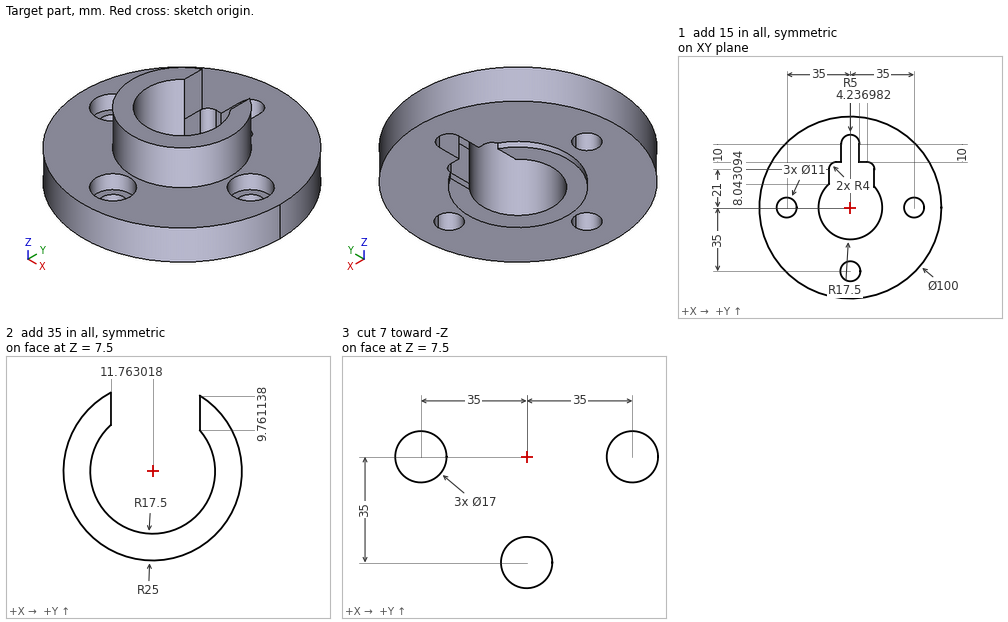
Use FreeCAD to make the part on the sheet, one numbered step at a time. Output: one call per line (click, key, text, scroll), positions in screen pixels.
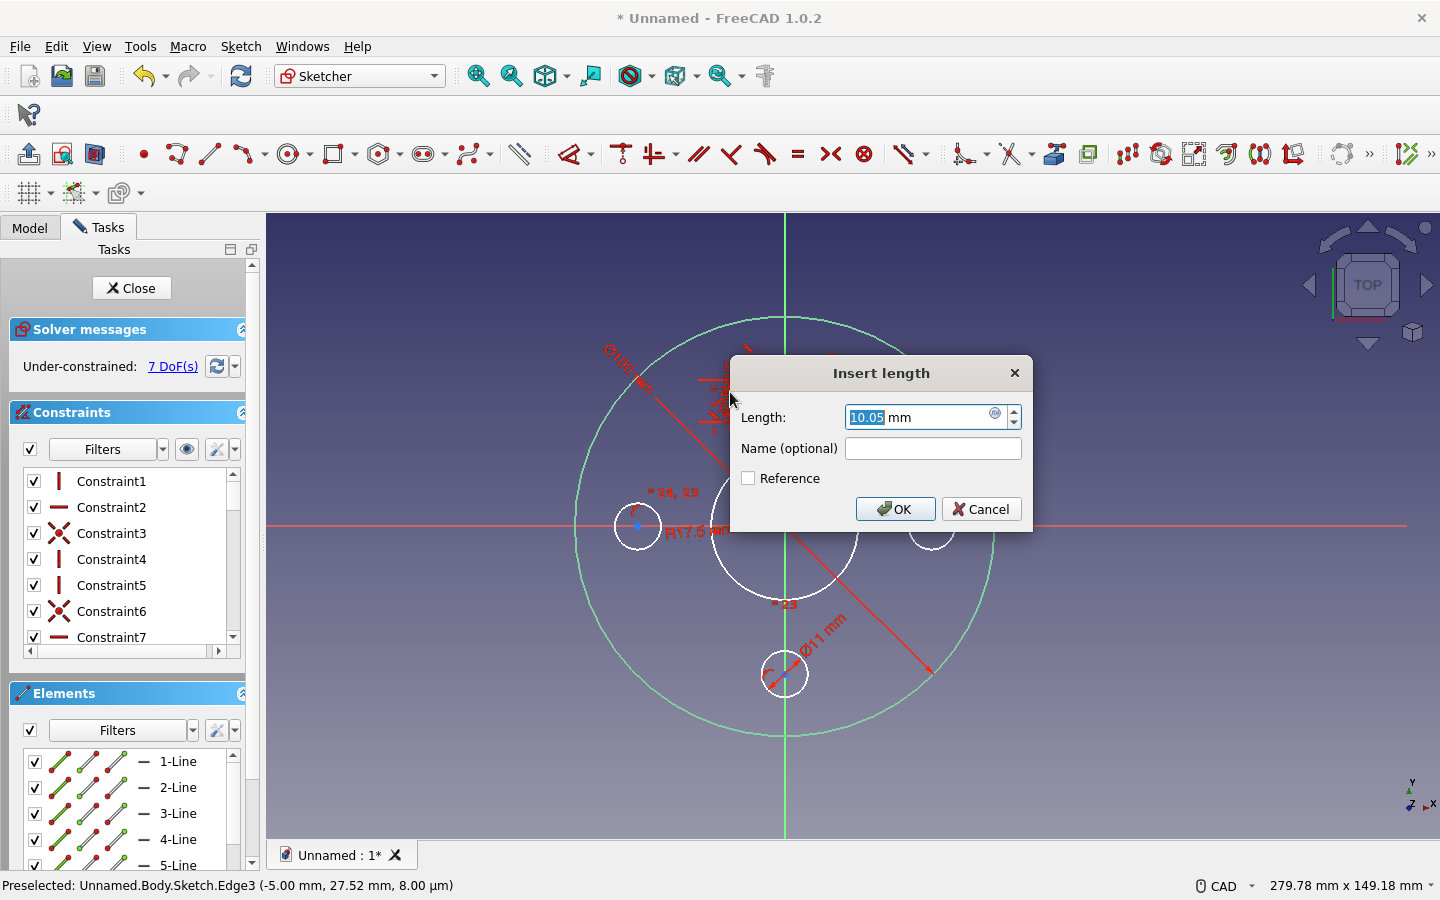
text(10)
key(Return)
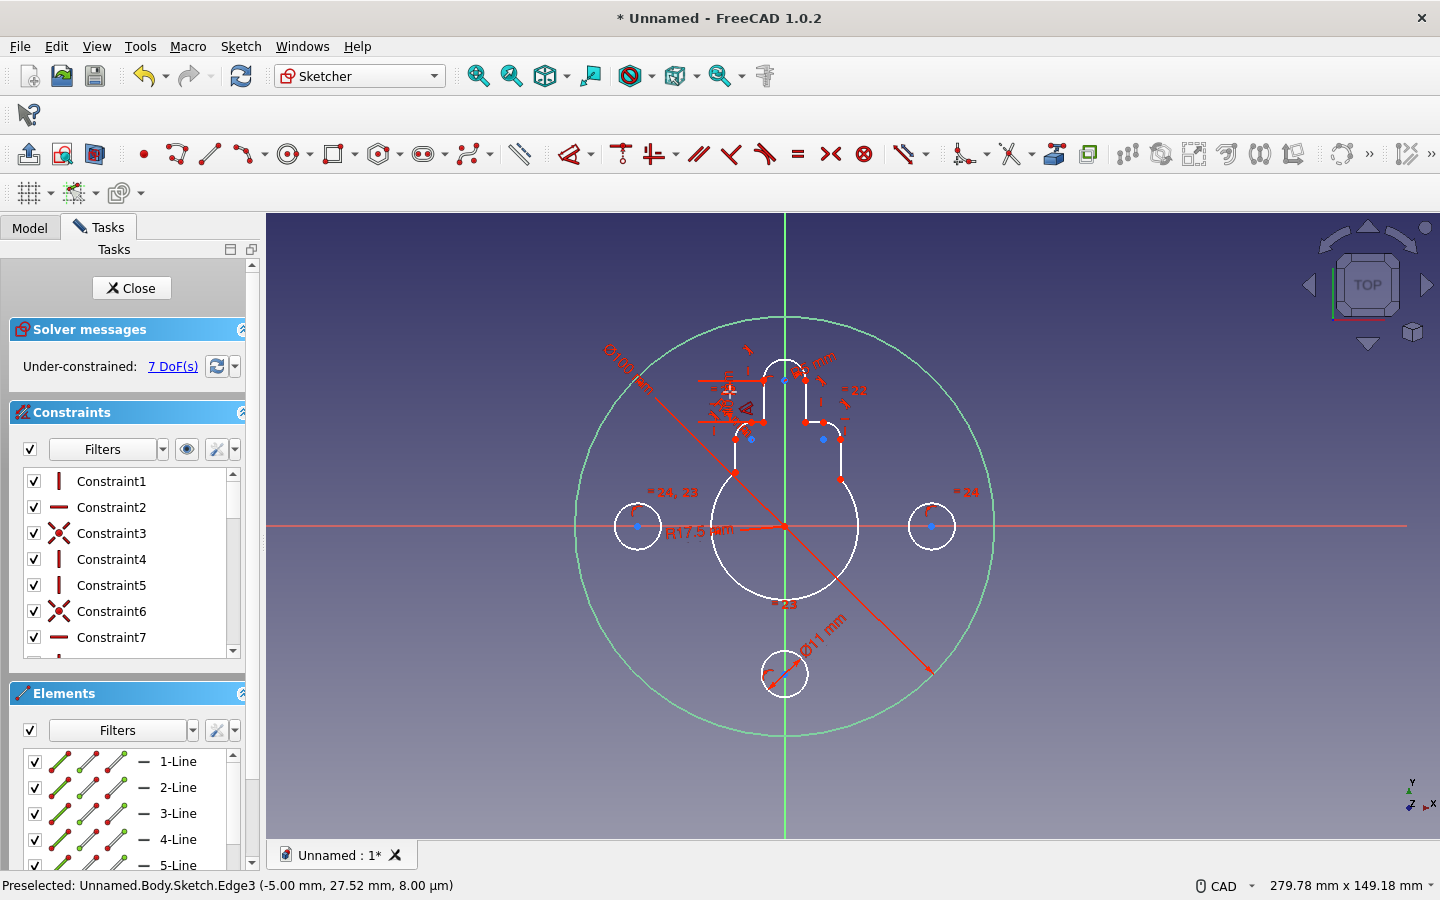
click(806, 393)
click(840, 401)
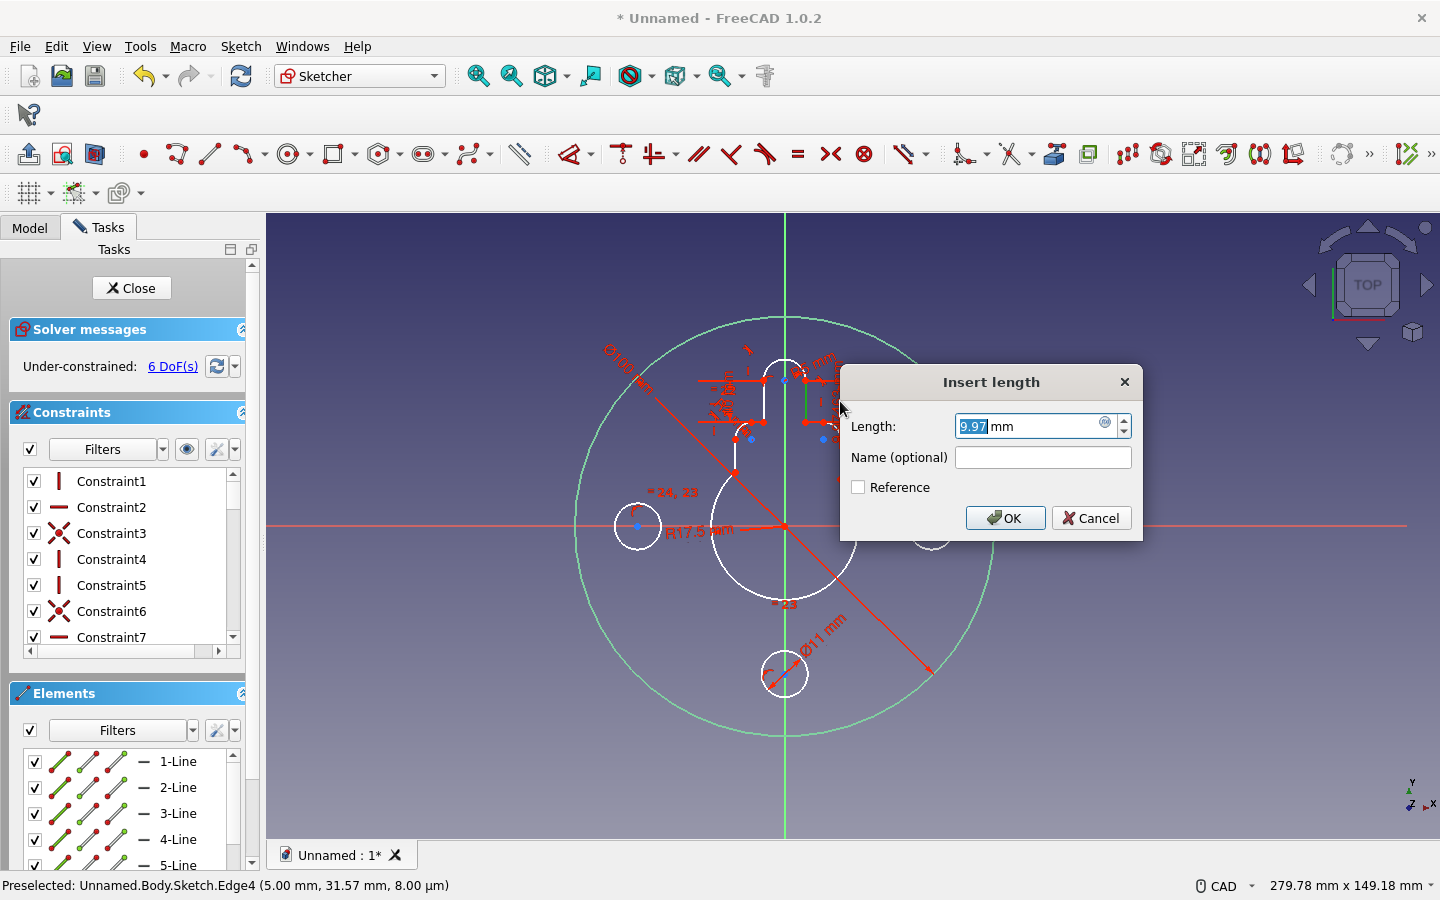
text(10)
key(Return)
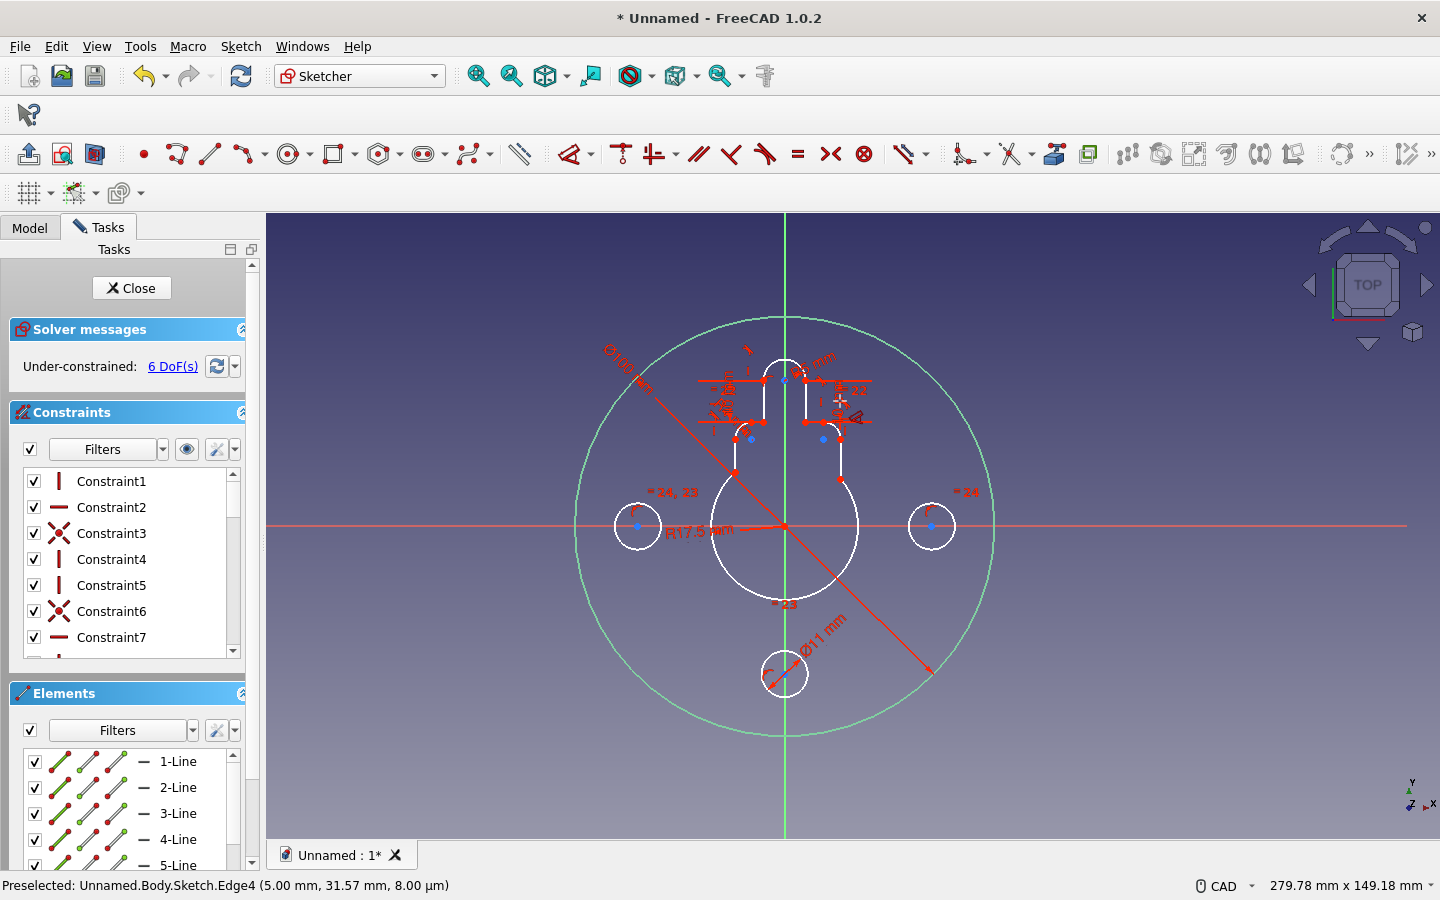
click(785, 674)
click(819, 566)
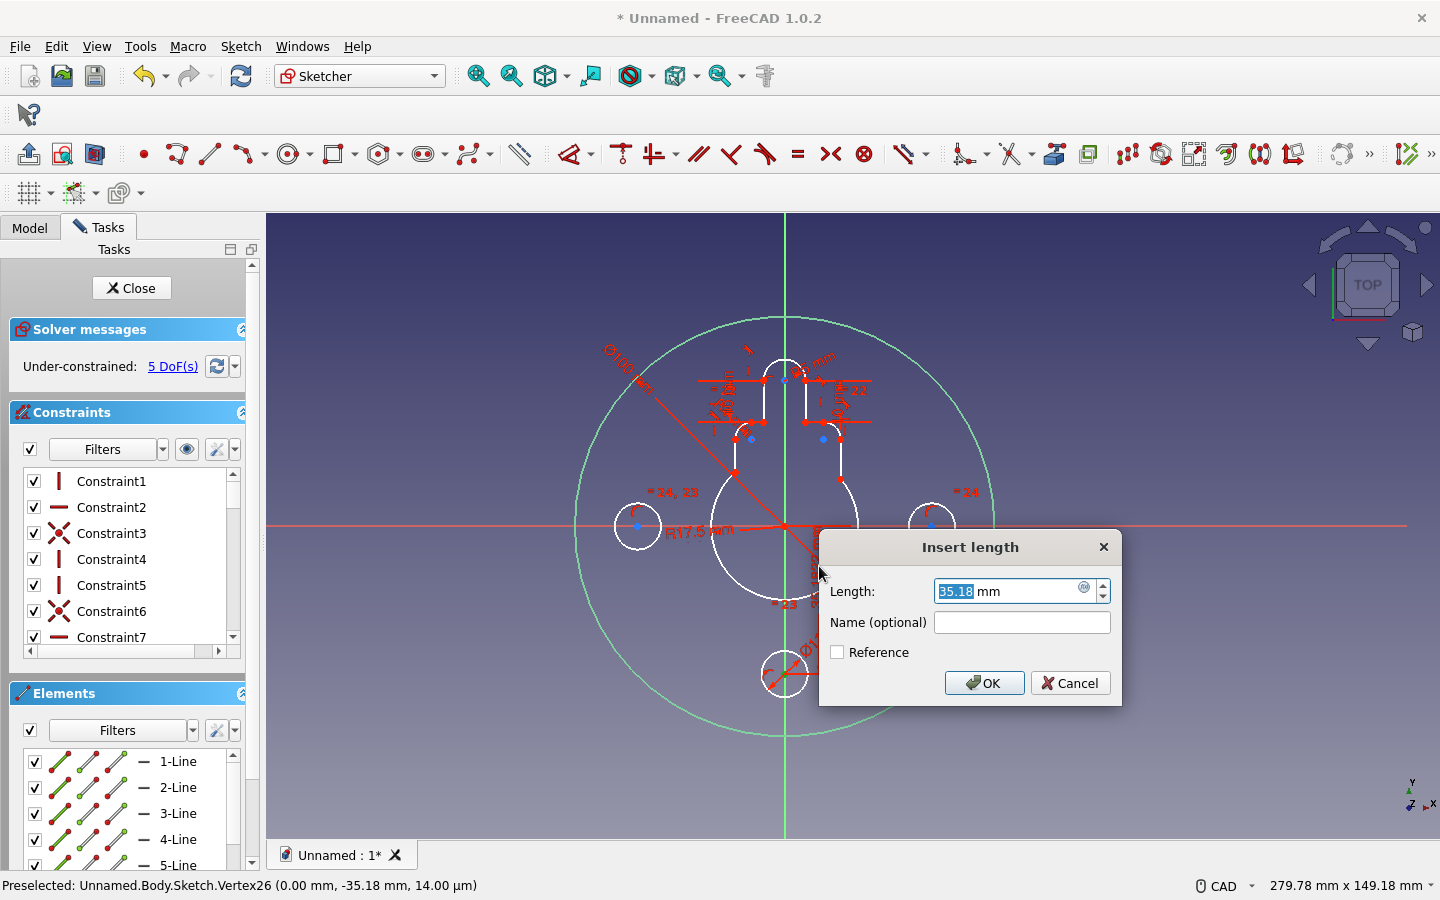
text(35)
key(Return)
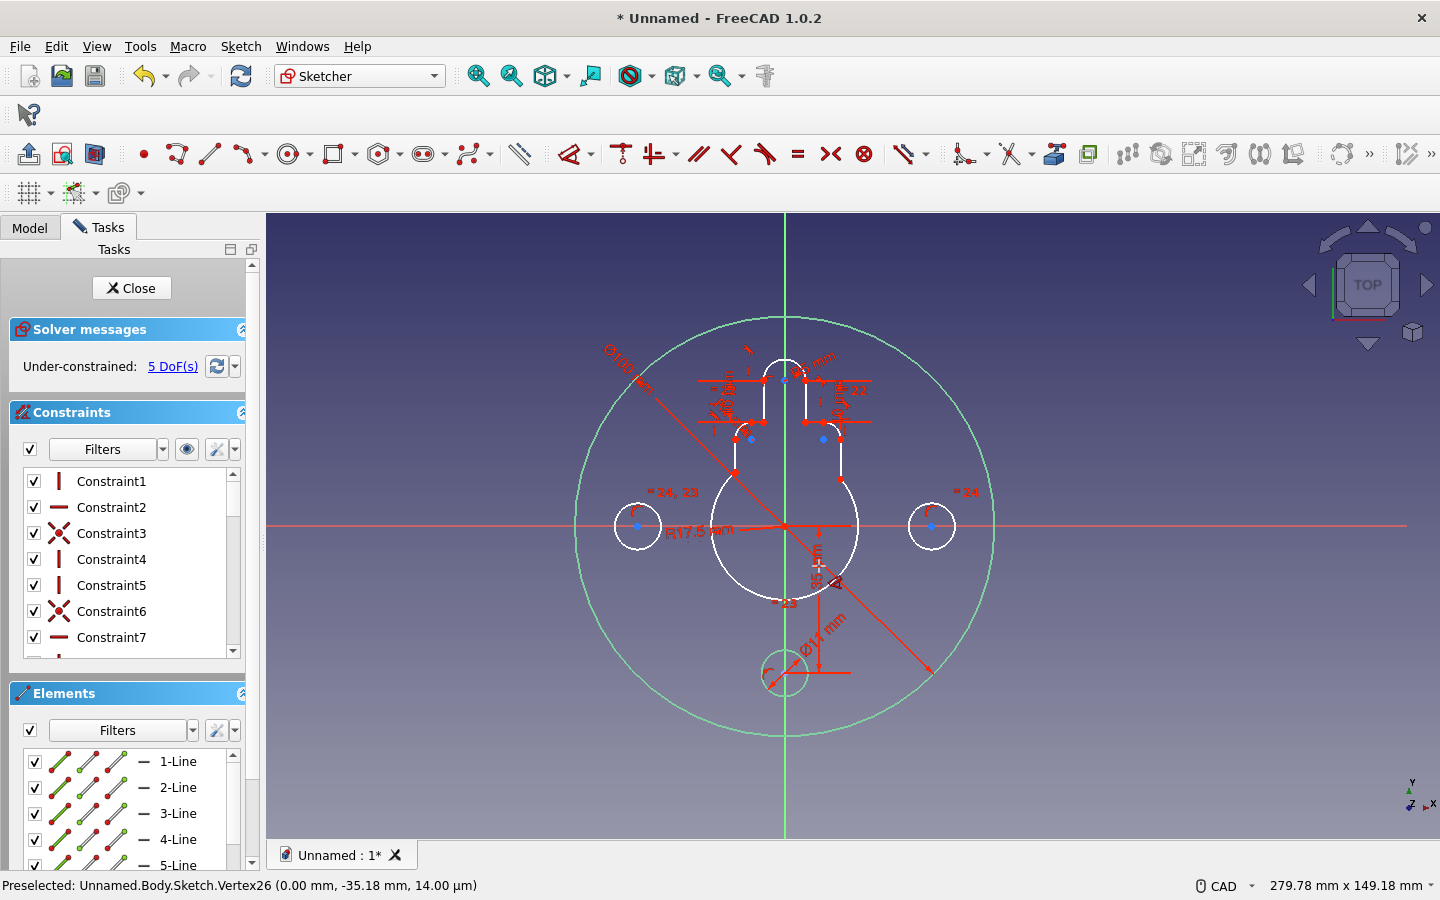
click(638, 526)
click(677, 560)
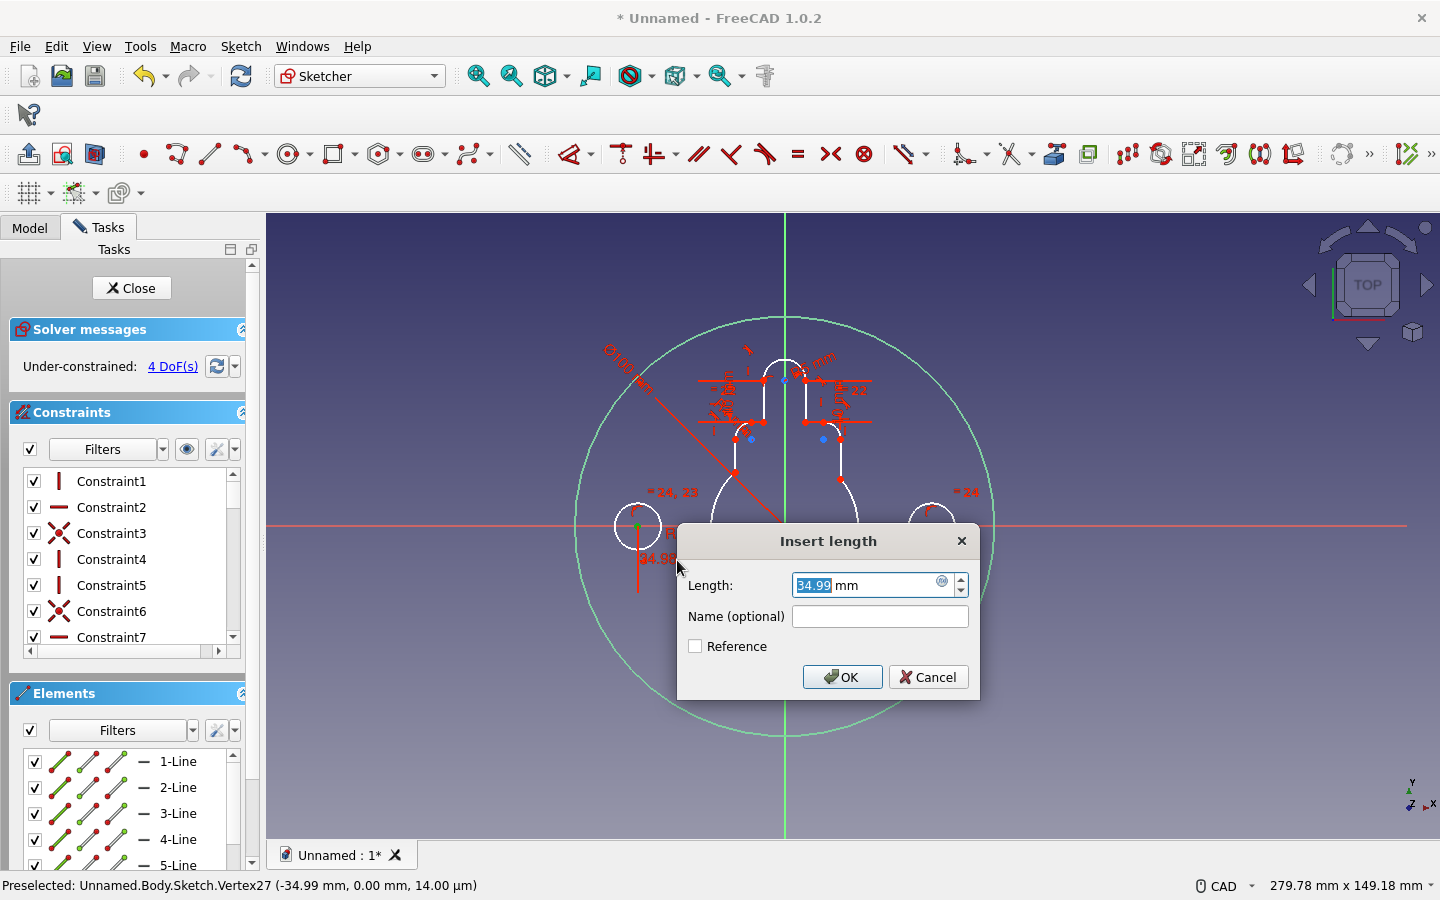
text(35)
key(Return)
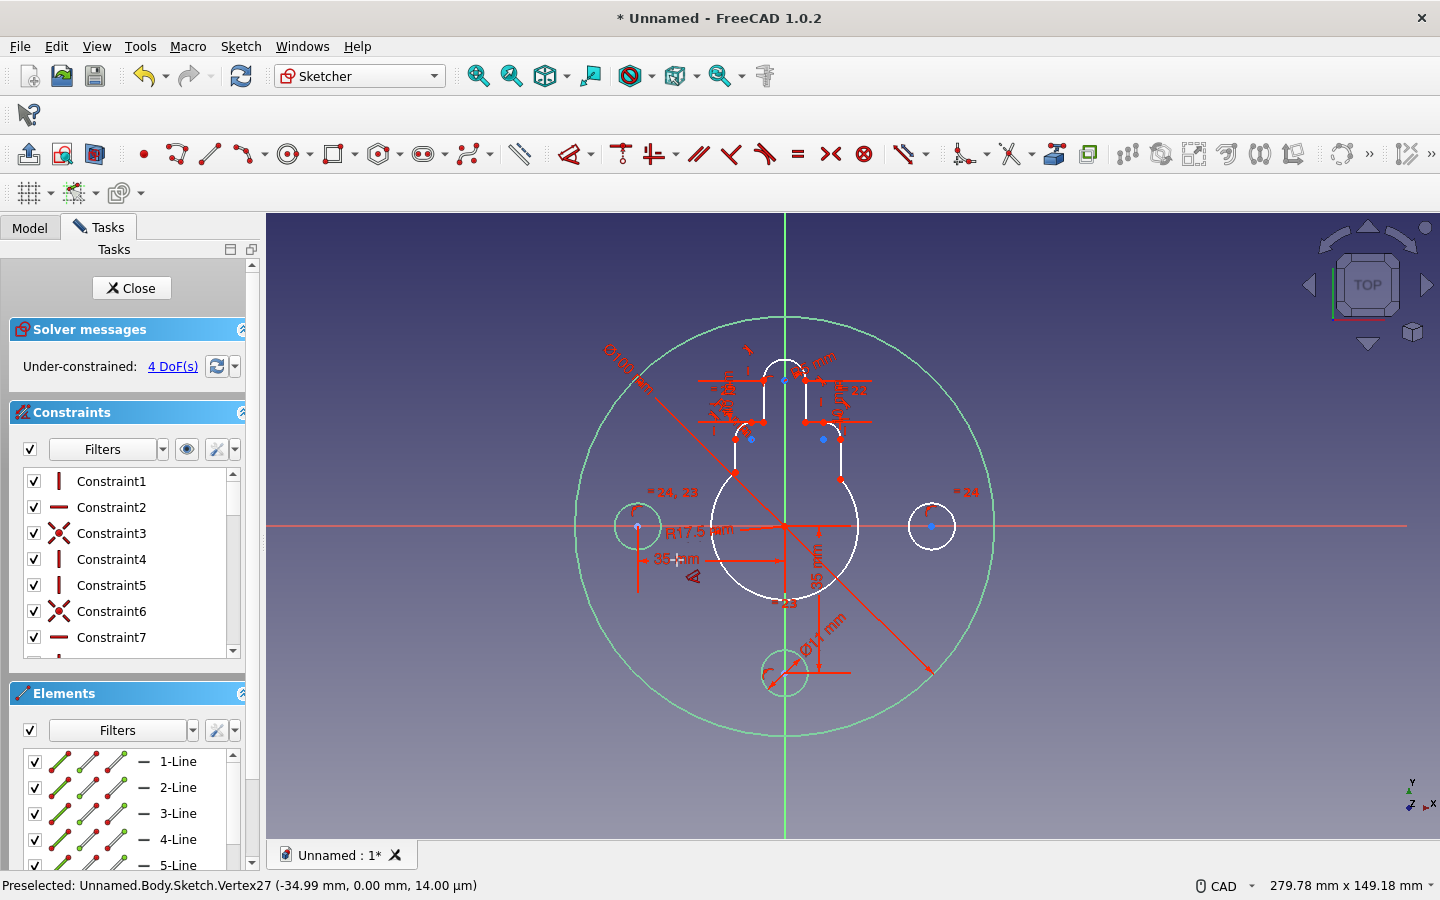
click(932, 526)
click(892, 560)